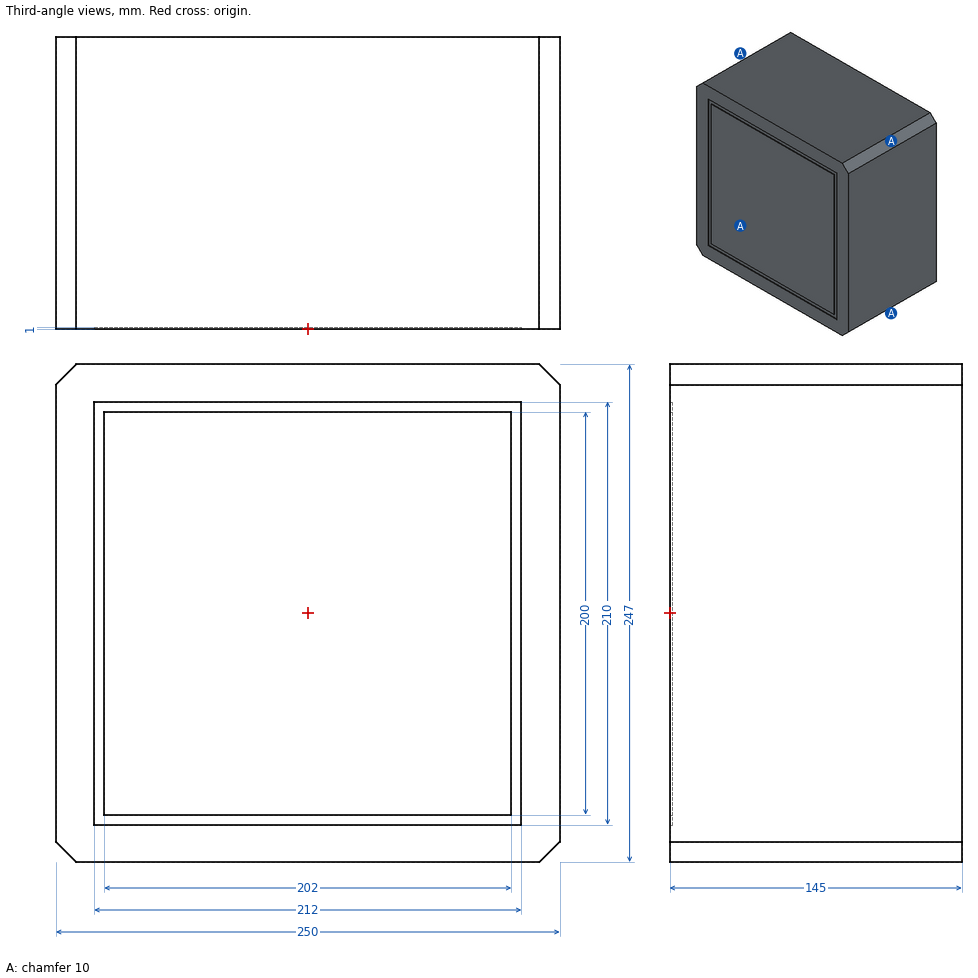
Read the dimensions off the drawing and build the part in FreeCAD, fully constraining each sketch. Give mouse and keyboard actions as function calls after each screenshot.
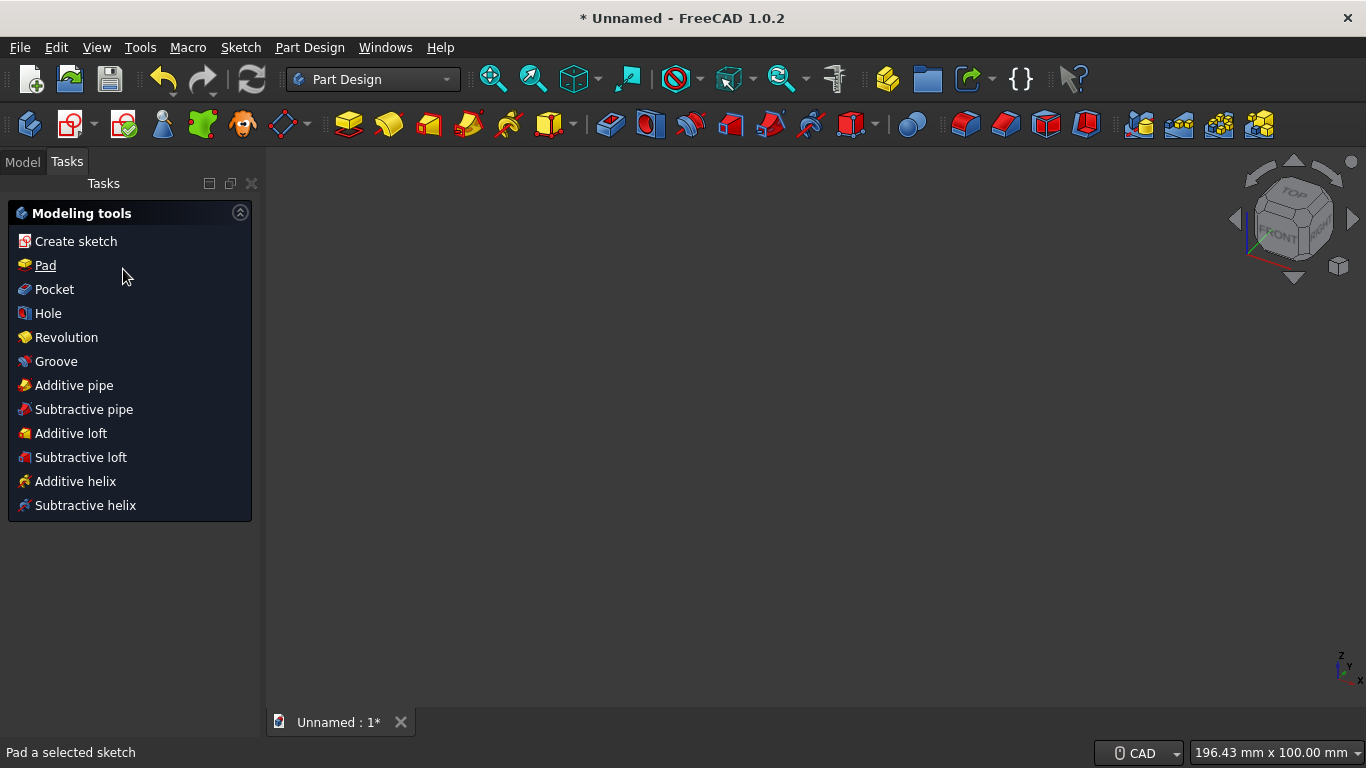
click(350, 124)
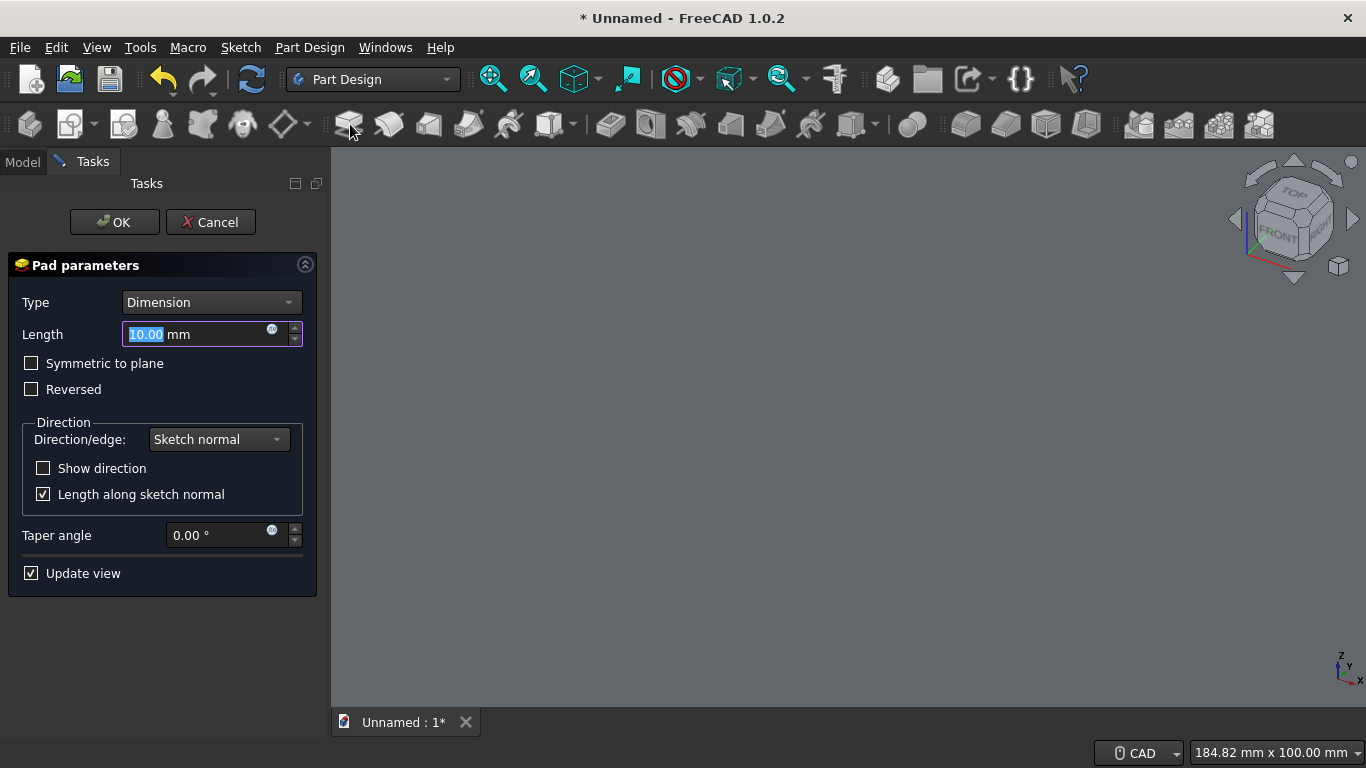
text(145)
key(Tab)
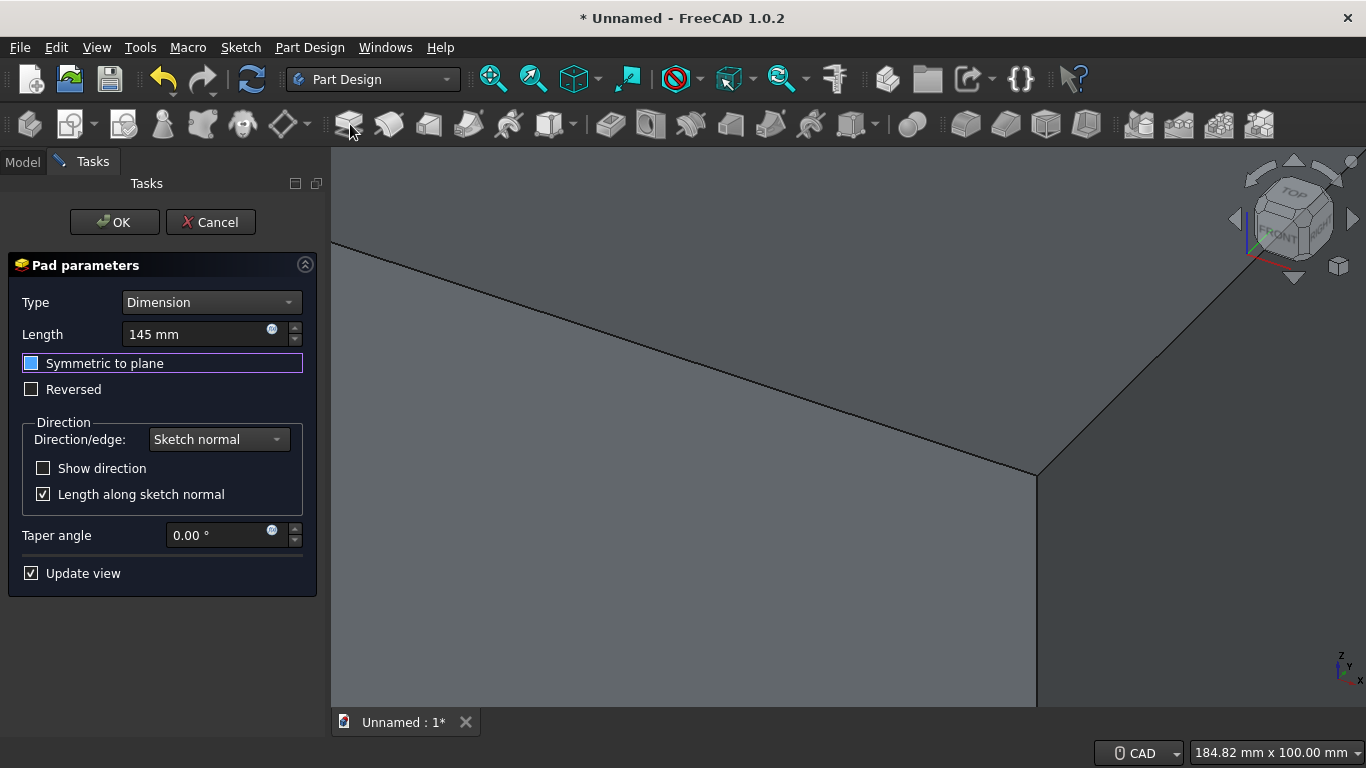
click(30, 389)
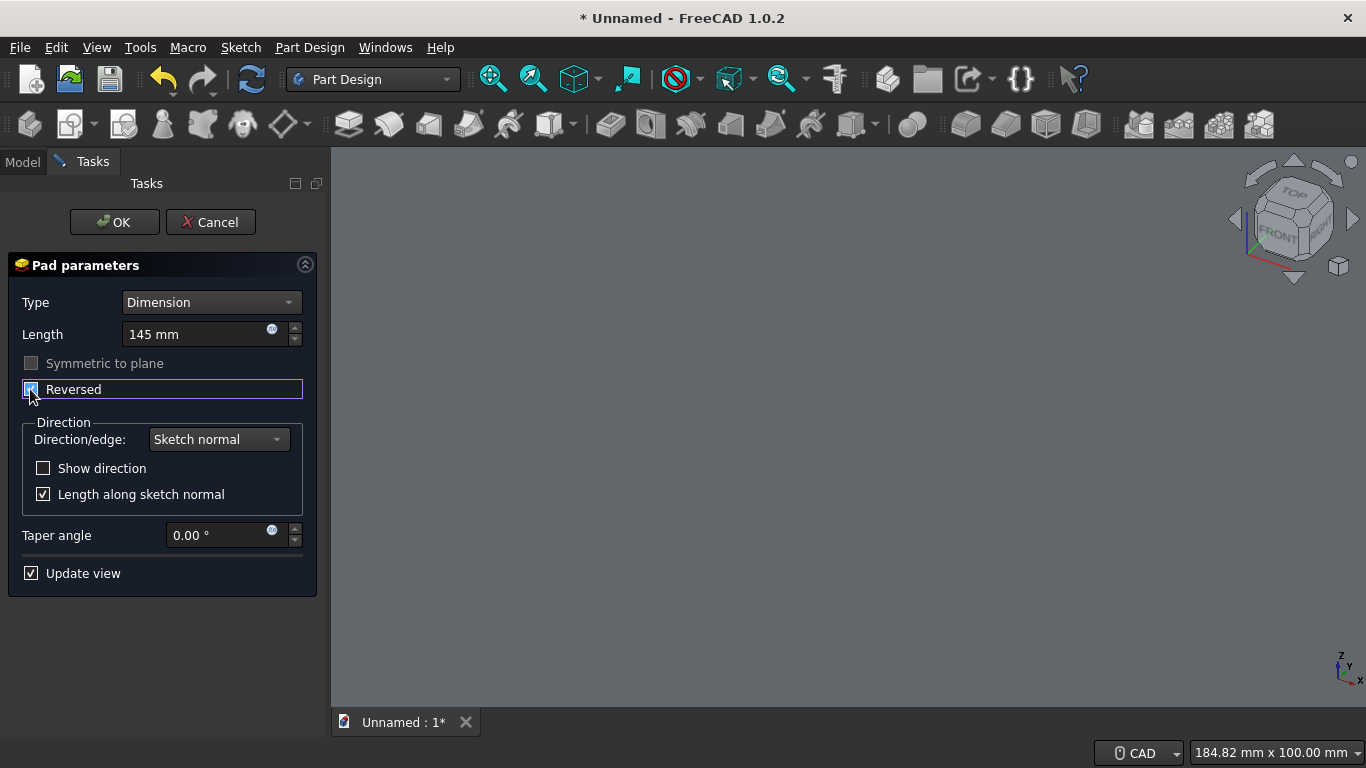
click(115, 222)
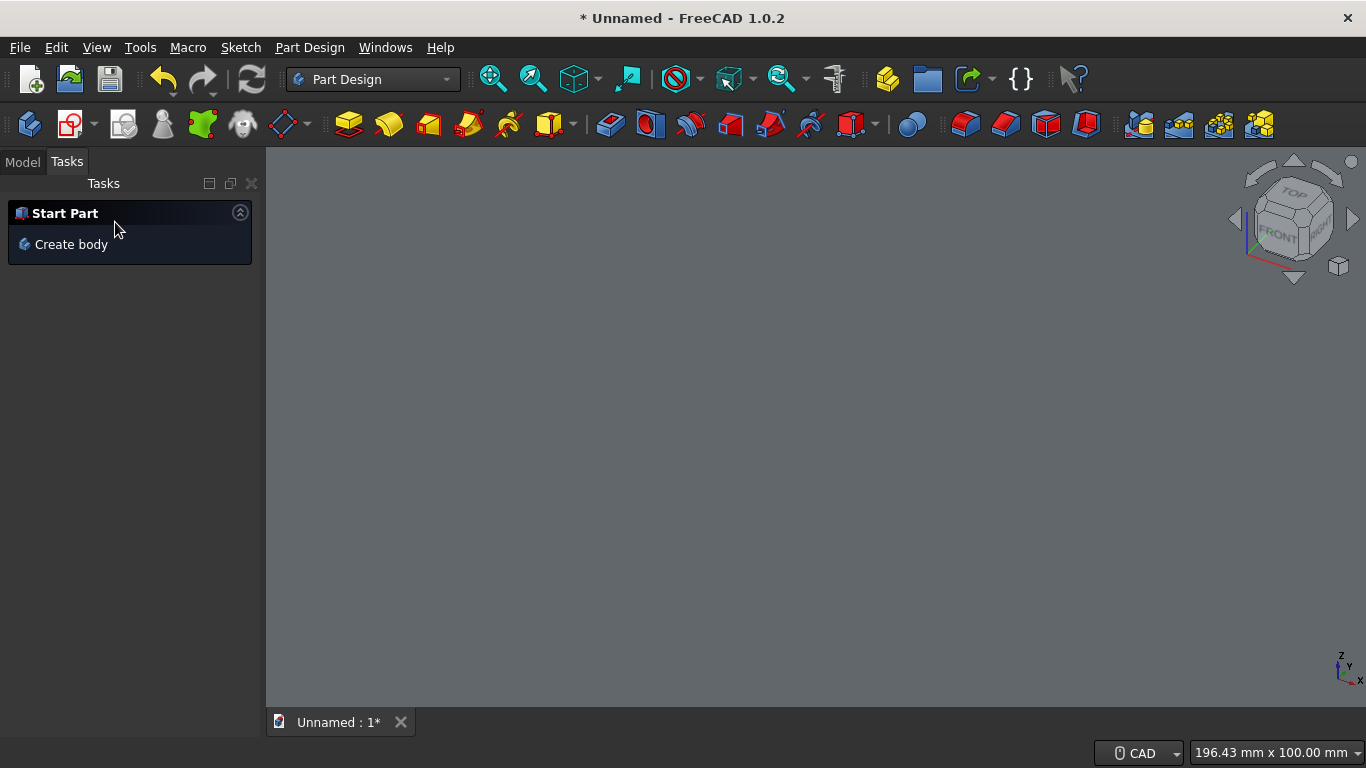
key(v)
key(f)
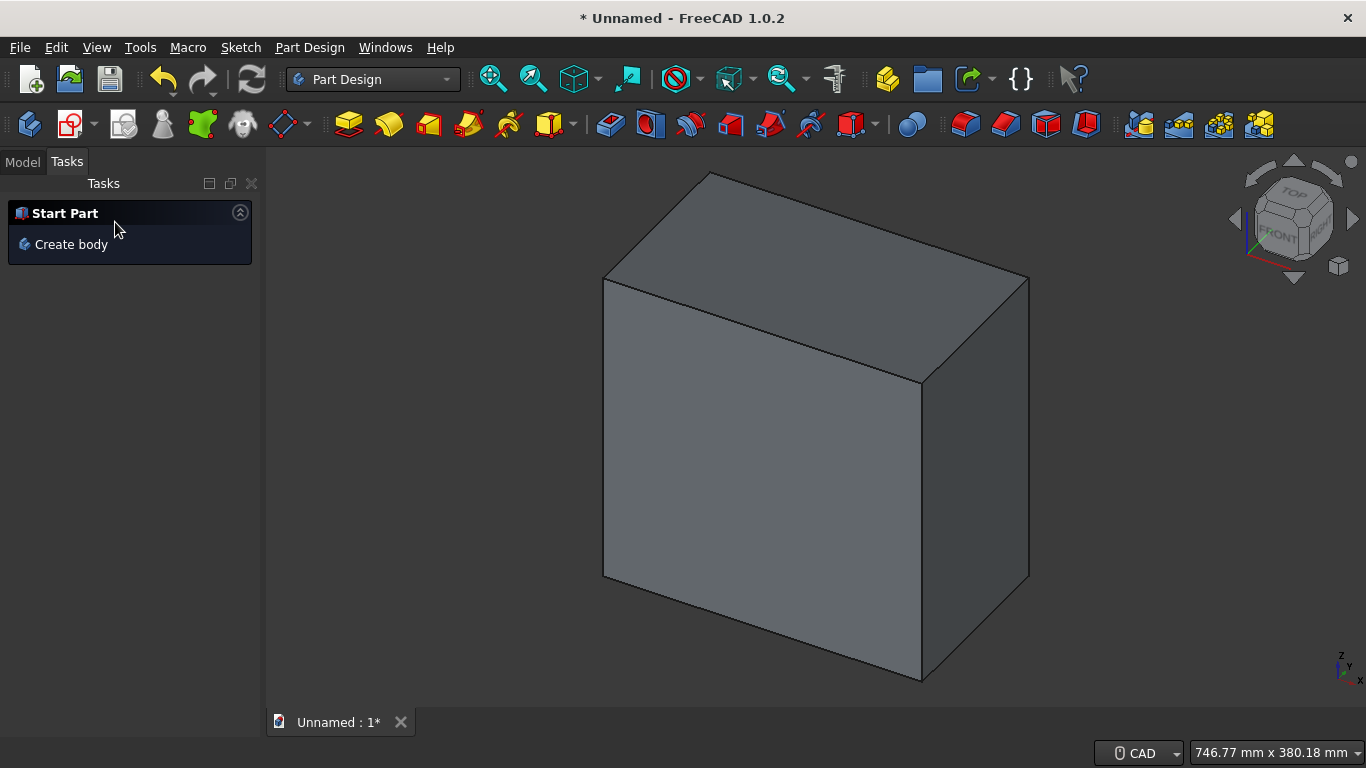
click(975, 330)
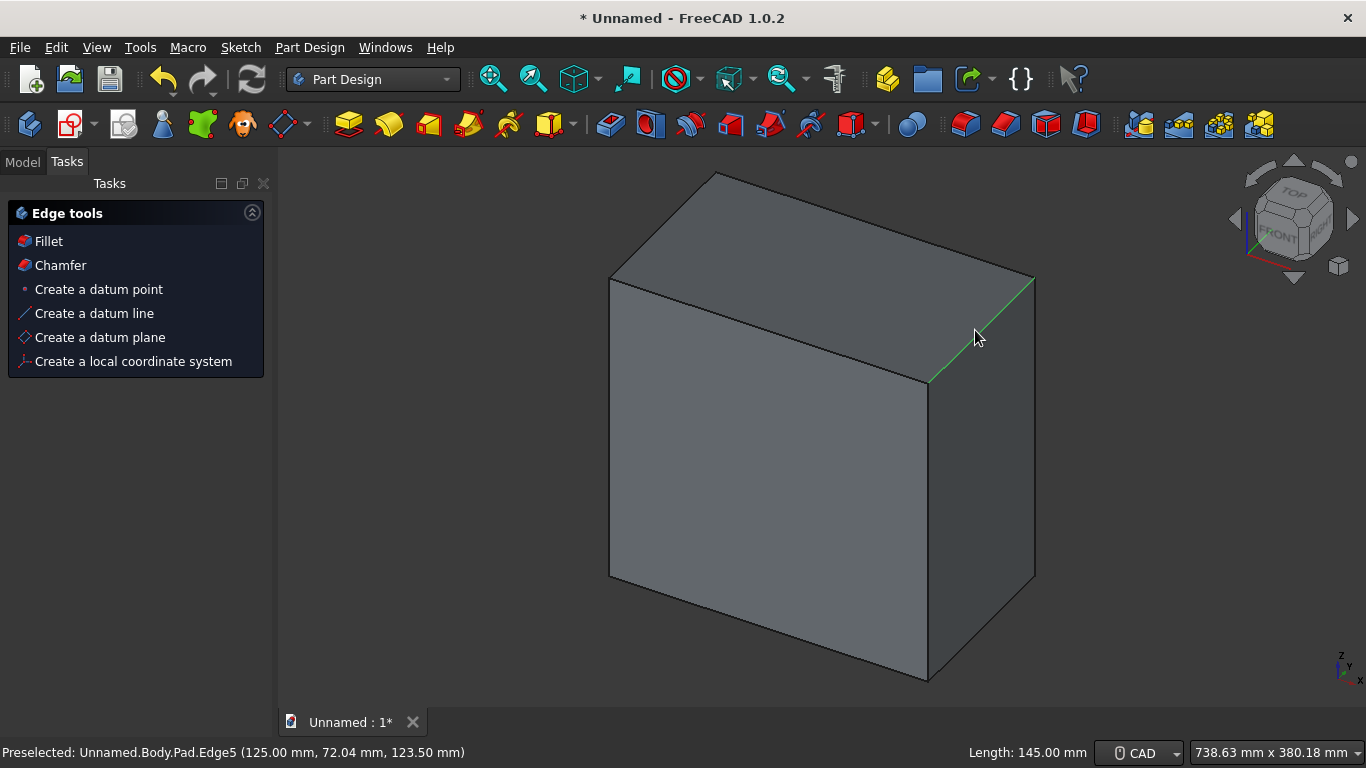
key(0)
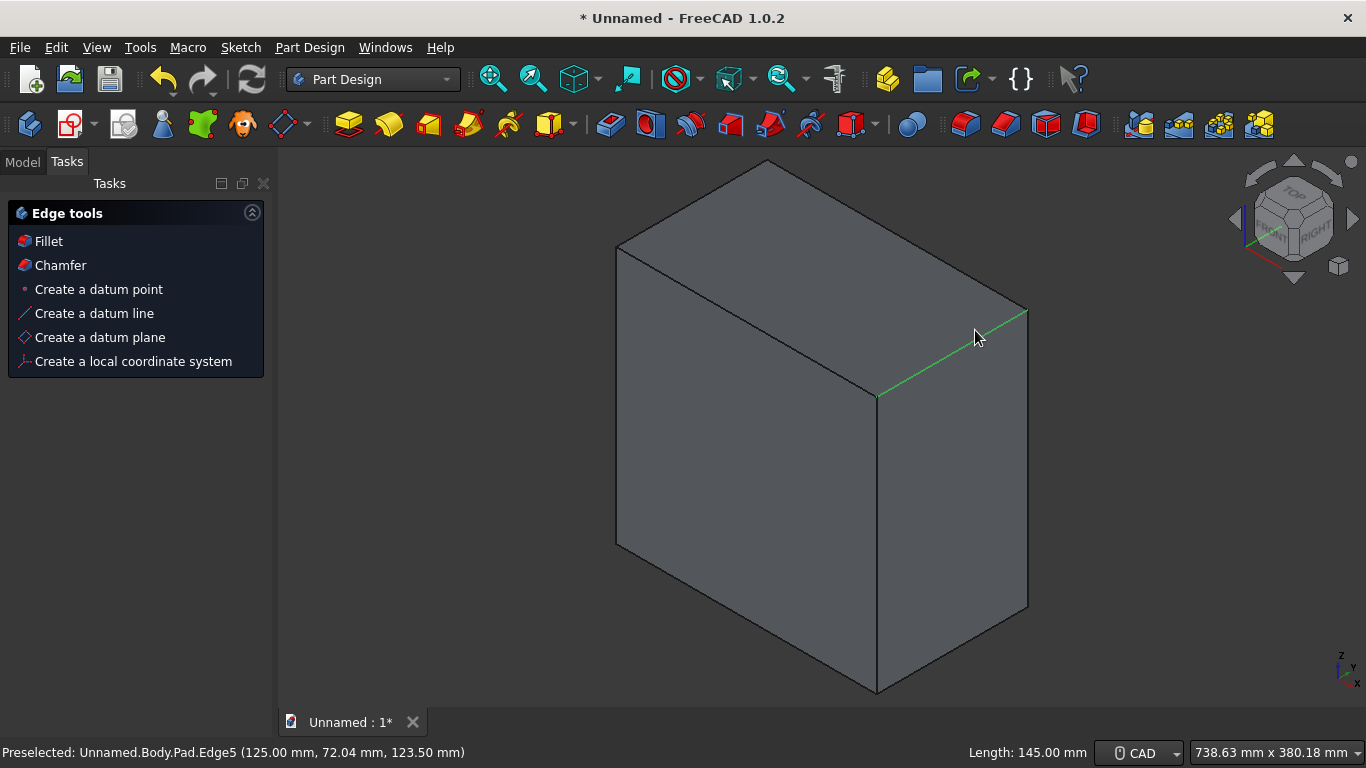
key(2)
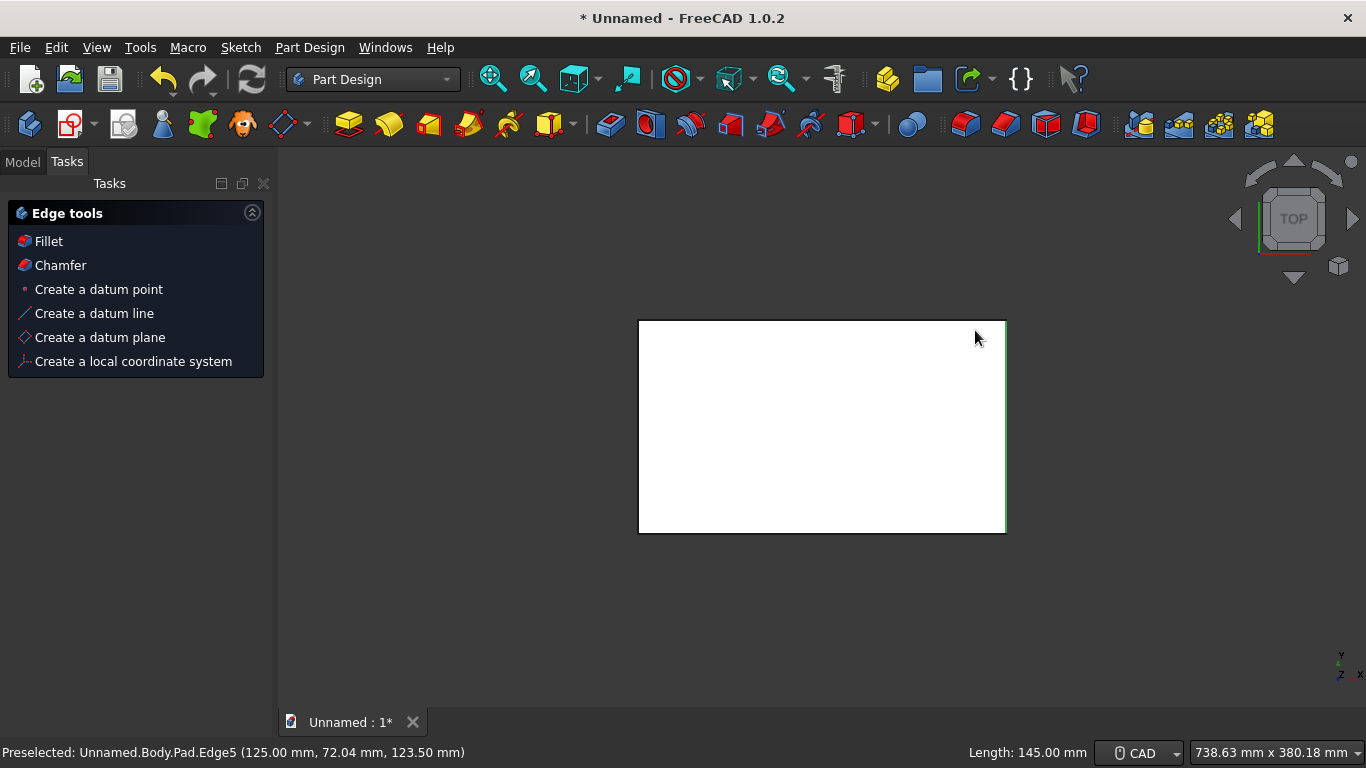
click(494, 80)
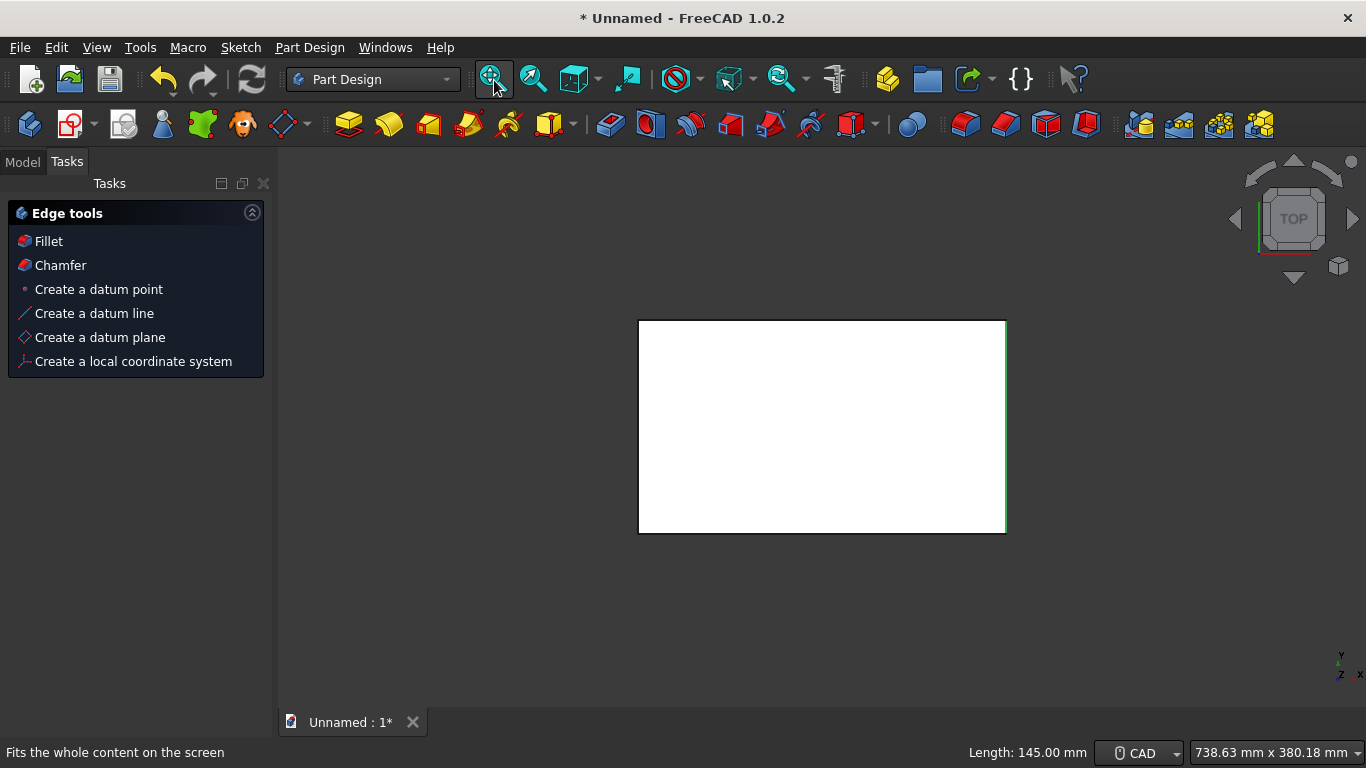
click(638, 426, ctrl)